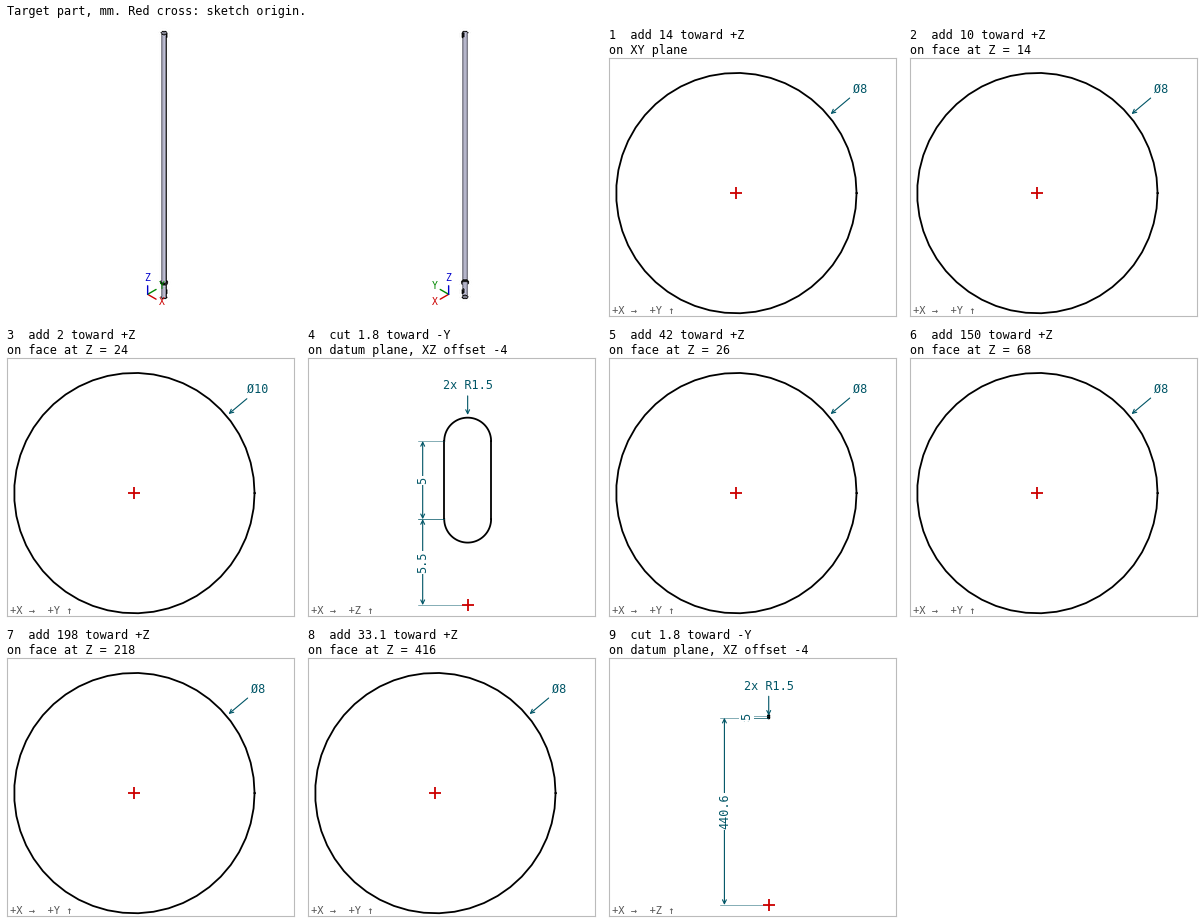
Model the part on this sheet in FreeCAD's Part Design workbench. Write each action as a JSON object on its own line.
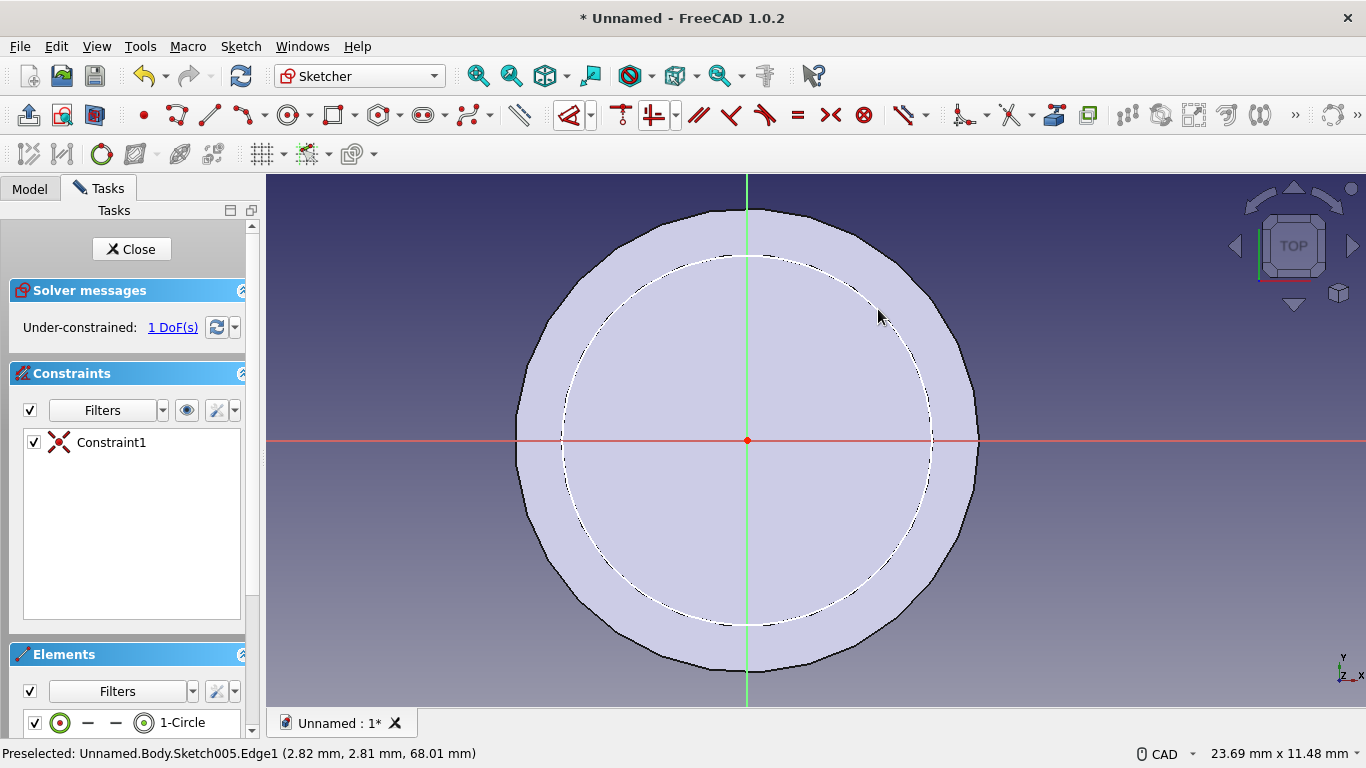
{"action": "left_click", "coordinate": [877, 309]}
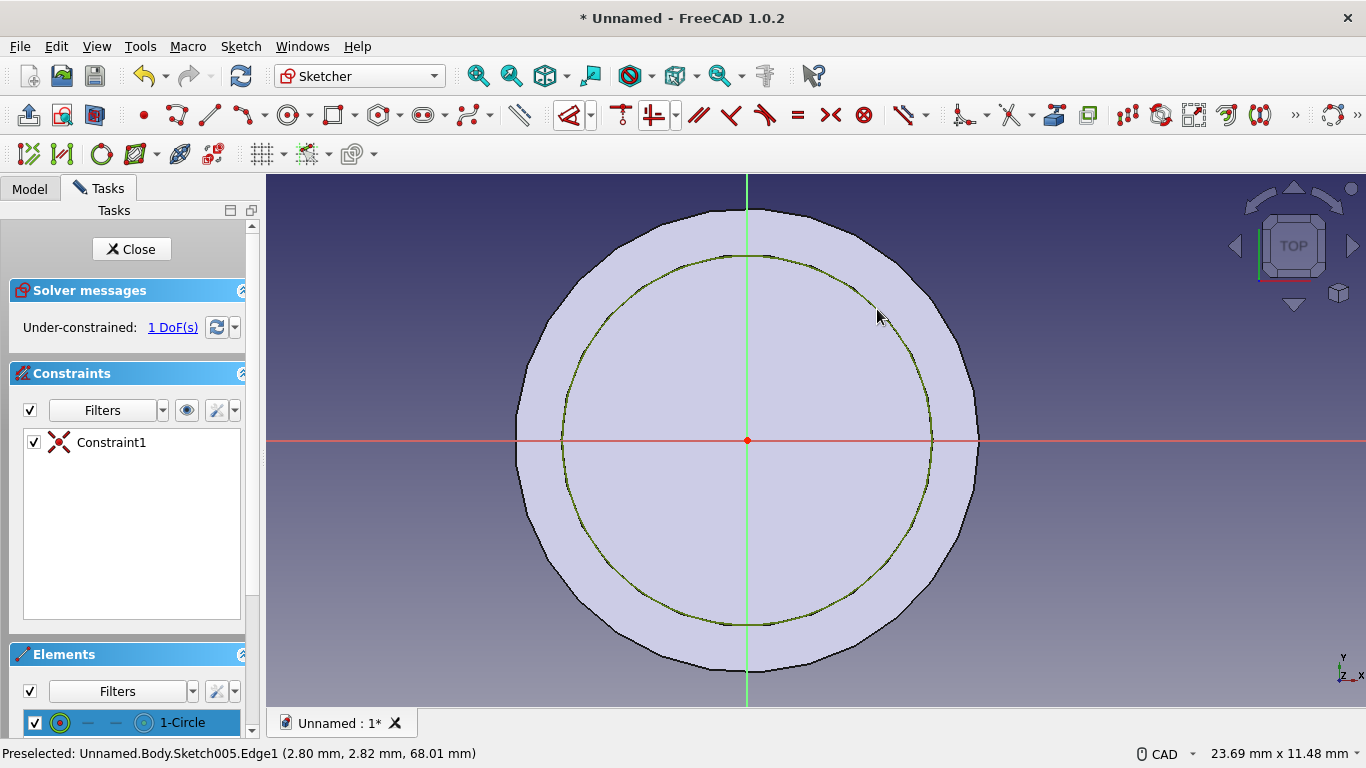
{"action": "key", "text": "k o"}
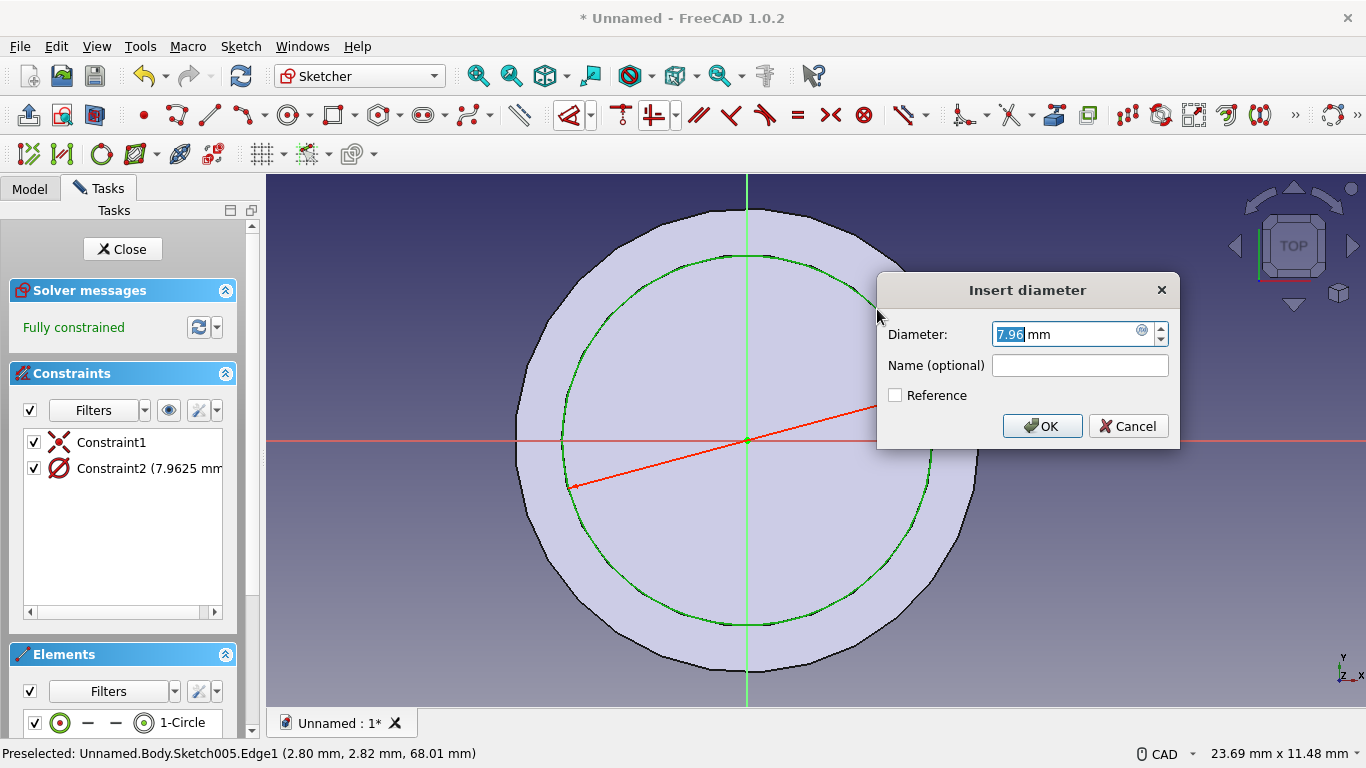
{"action": "type", "text": "8"}
{"action": "key", "text": "Return"}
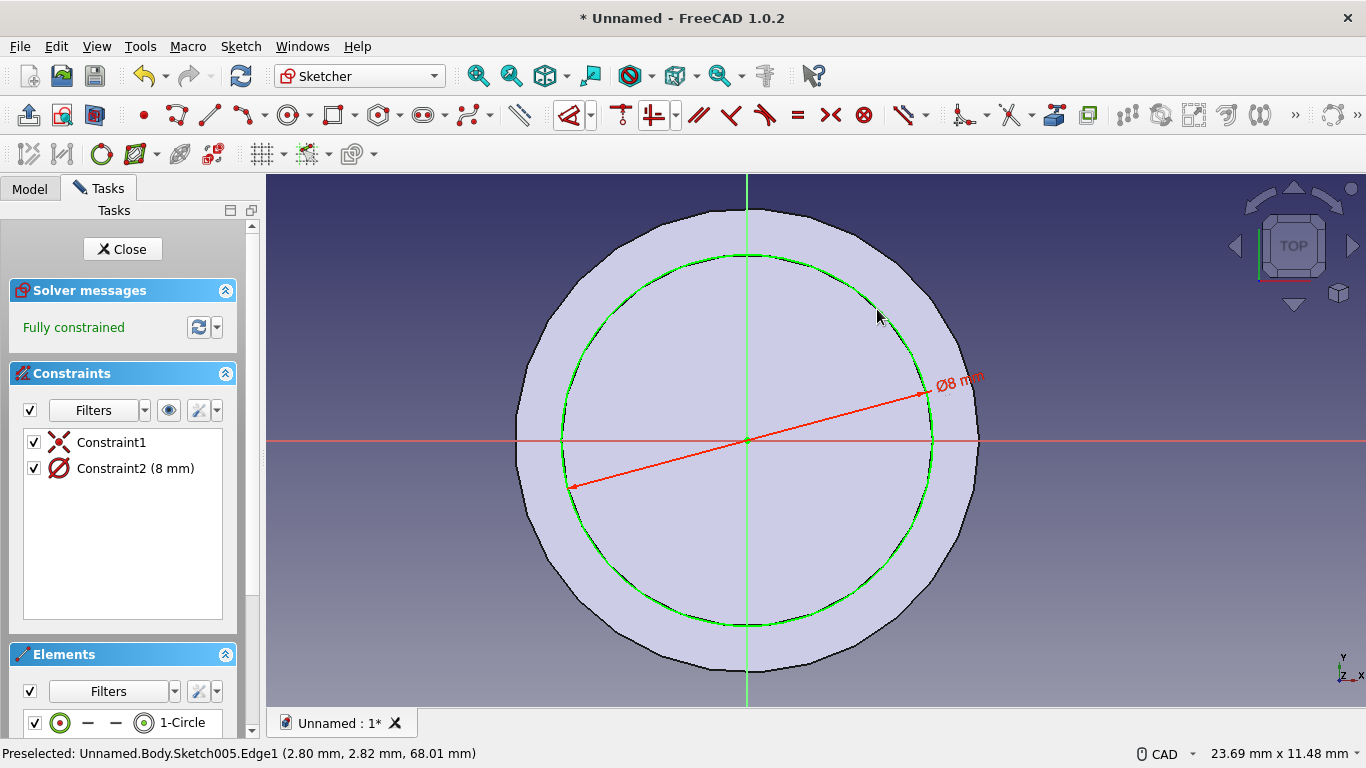
{"action": "left_click", "coordinate": [123, 249]}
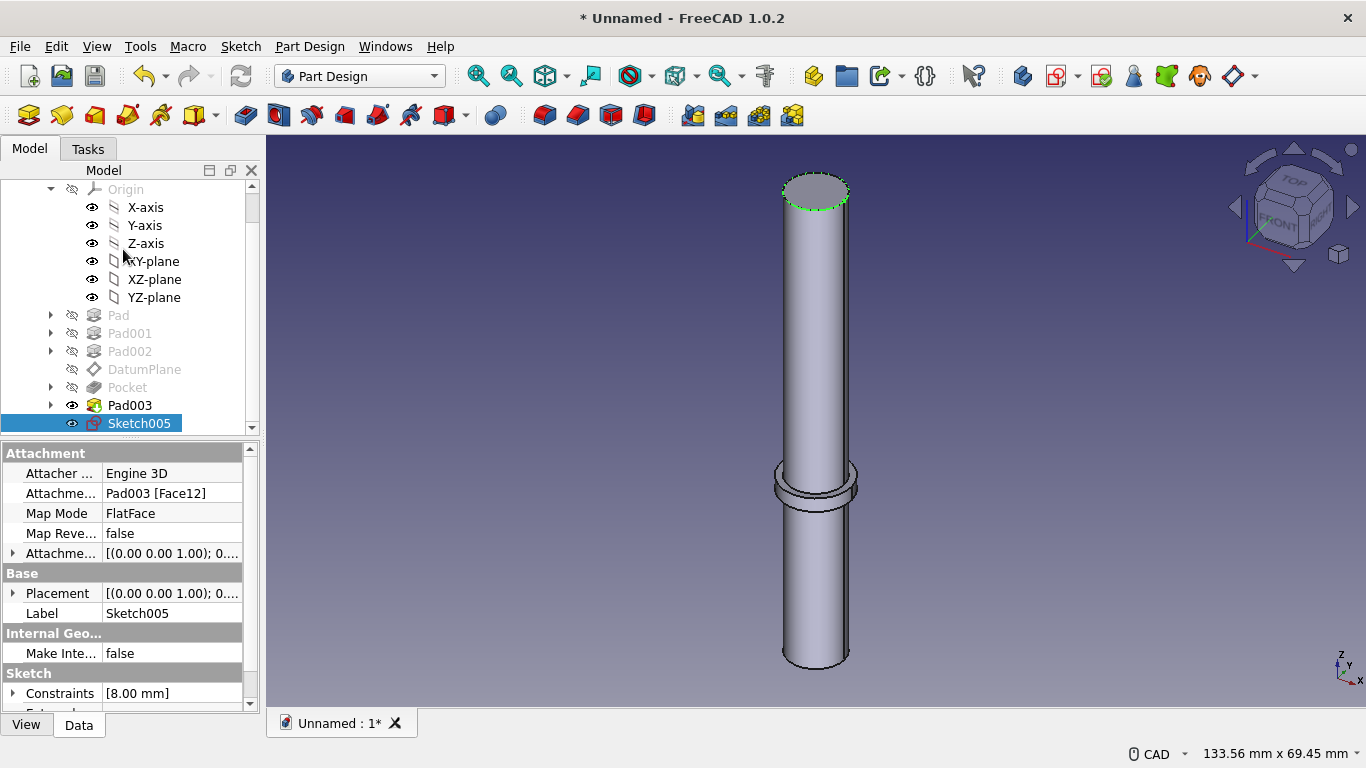
{"action": "left_click", "coordinate": [29, 116]}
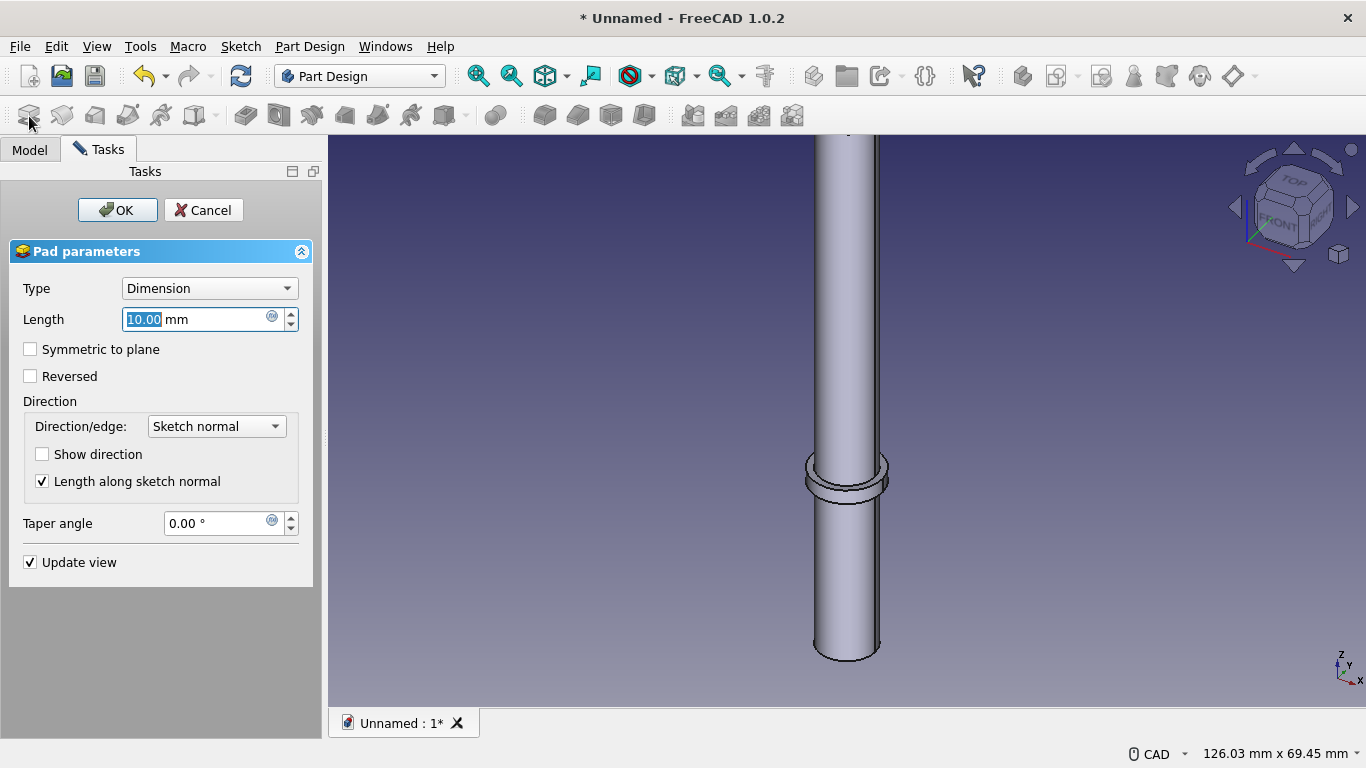
{"action": "type", "text": "150"}
{"action": "key", "text": "Tab"}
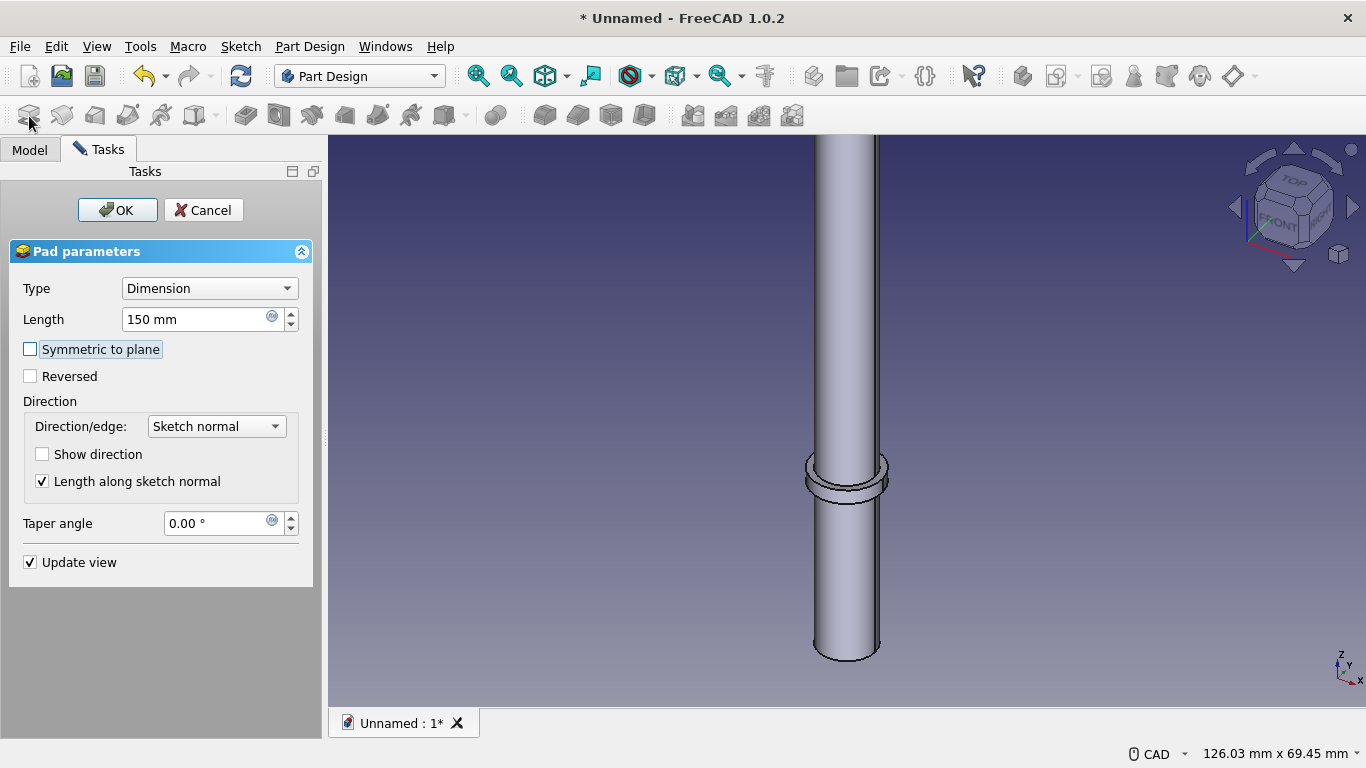
{"action": "left_click", "coordinate": [118, 210]}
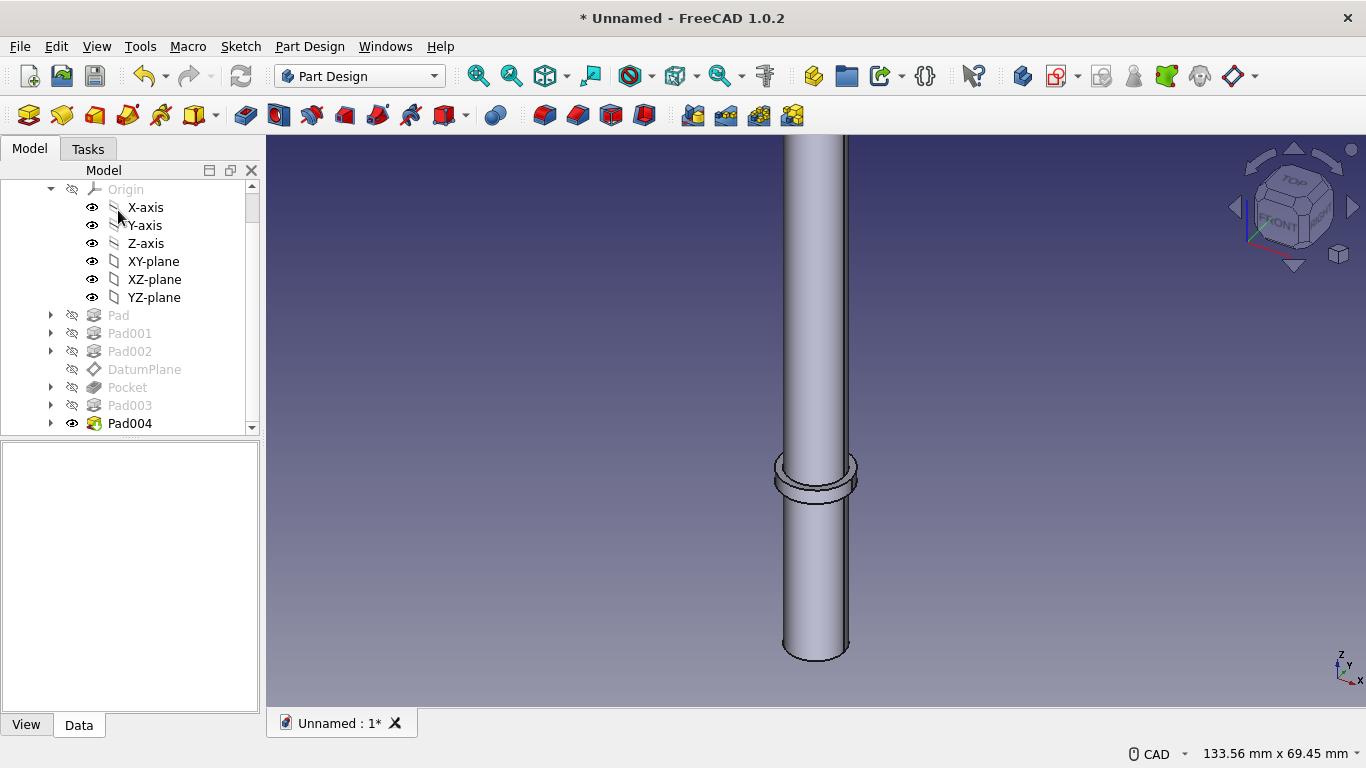
{"action": "left_click", "coordinate": [479, 76]}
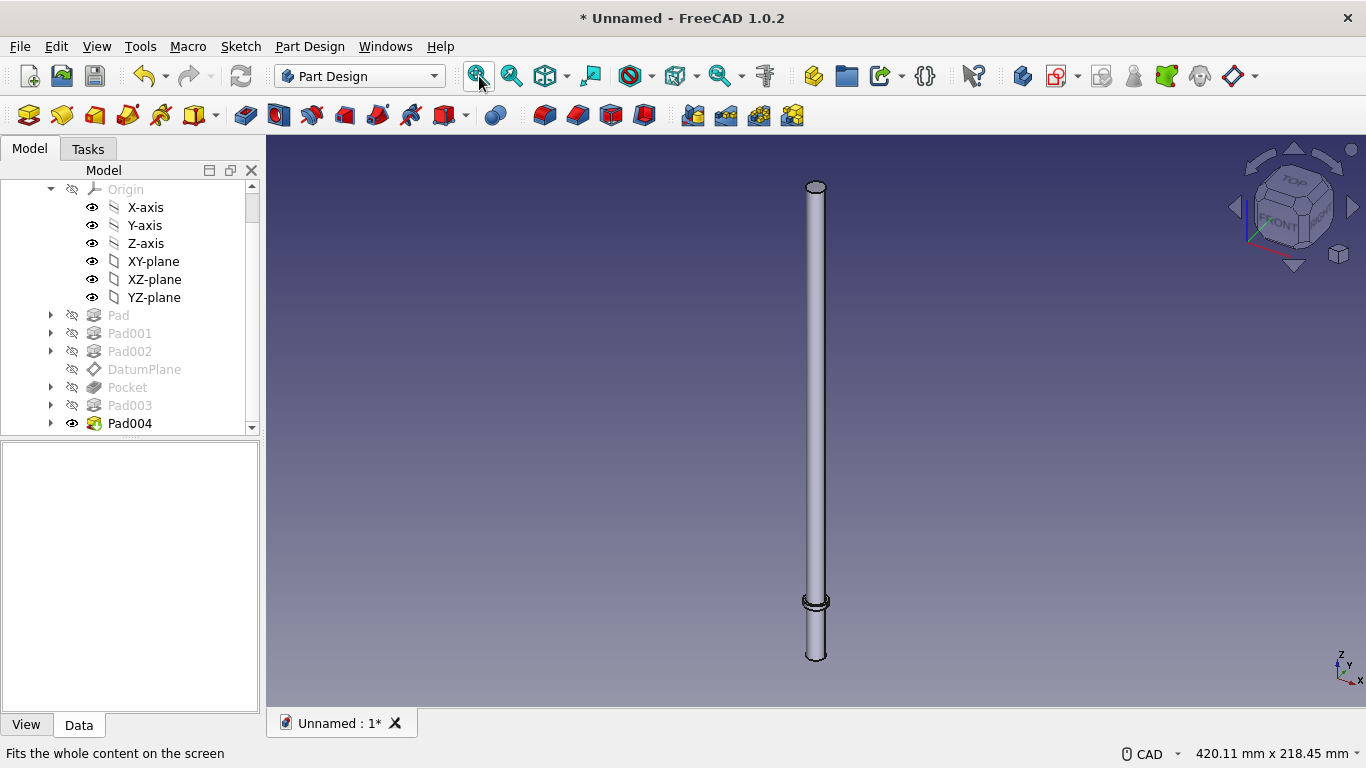
{"action": "key", "text": "0"}